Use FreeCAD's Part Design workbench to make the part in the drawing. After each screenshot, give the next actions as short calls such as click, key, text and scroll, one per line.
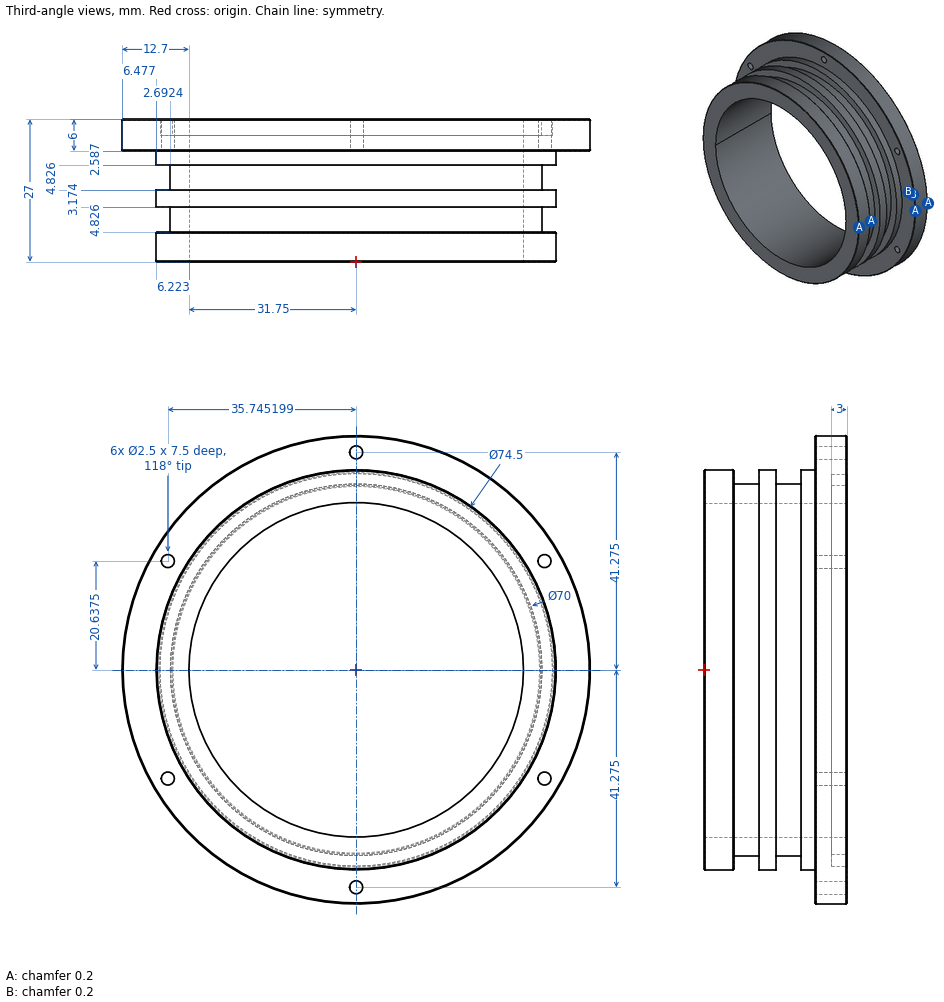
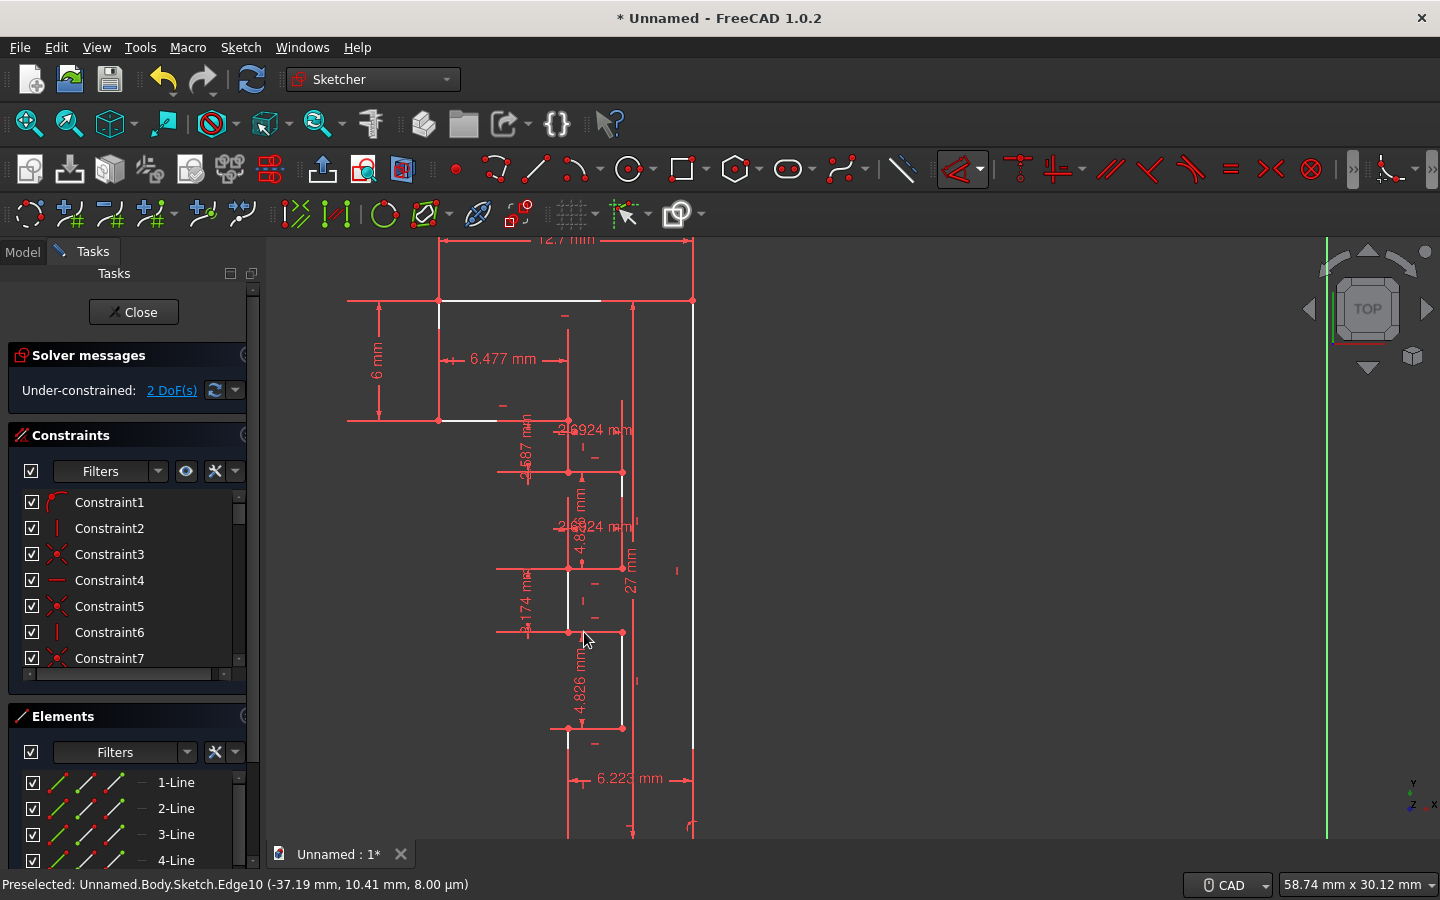
key(l)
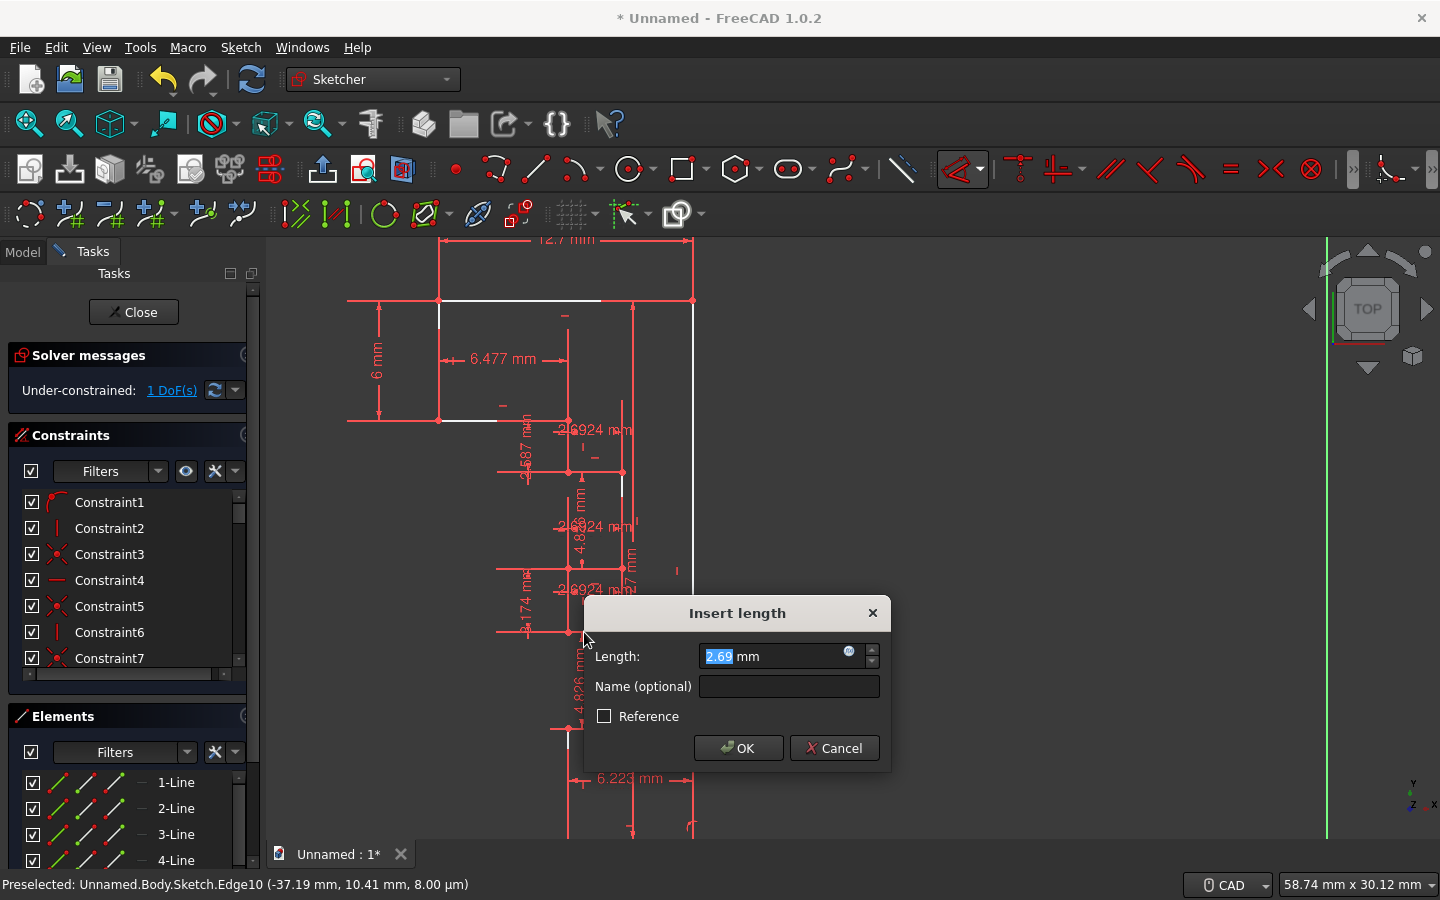
text(2.6924)
key(Return)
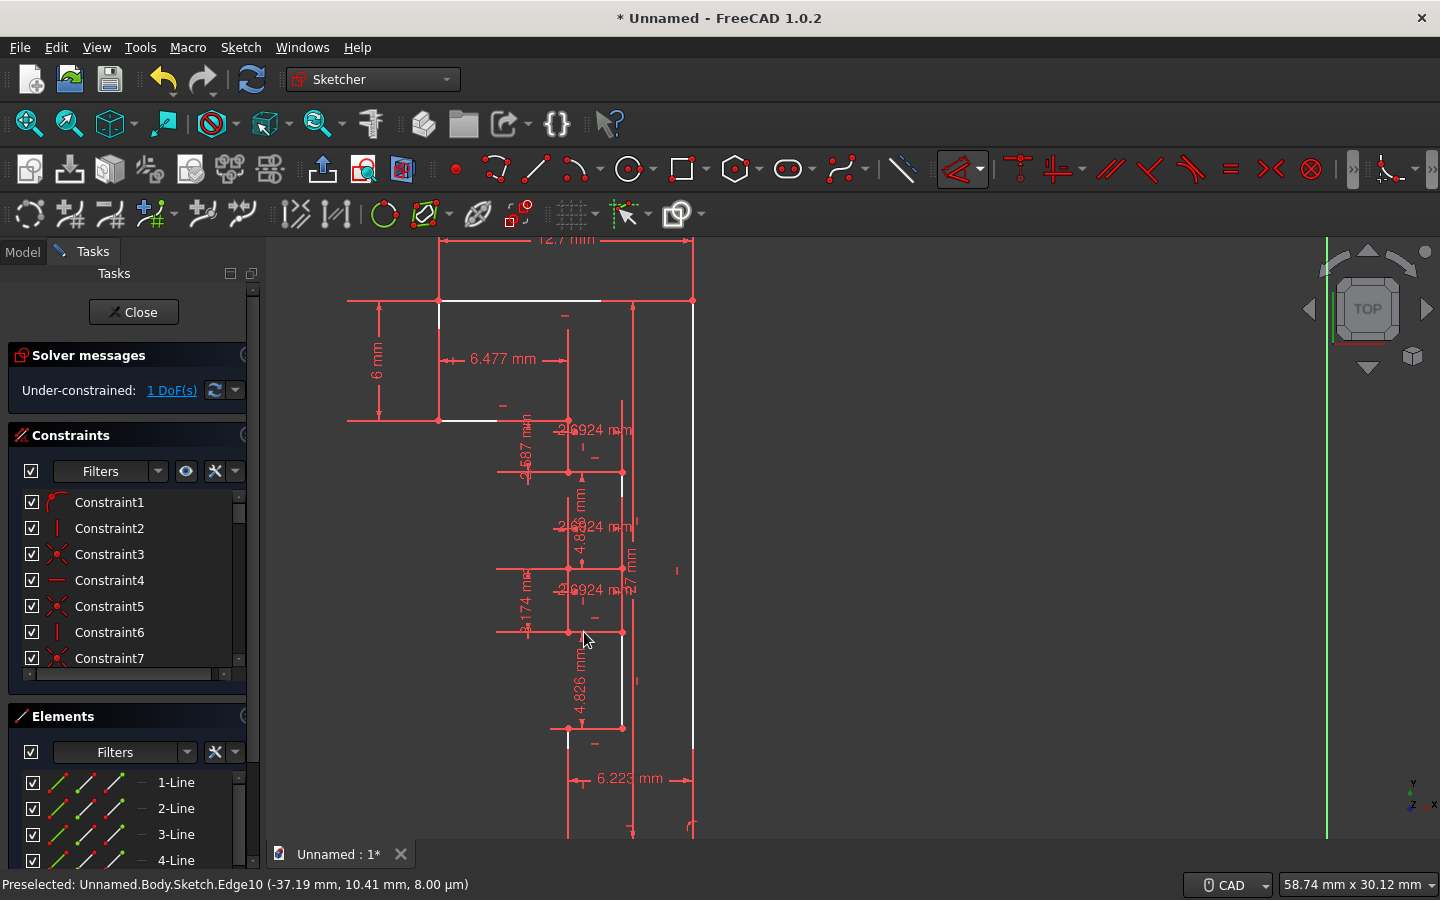
scroll(584, 472, down, 2)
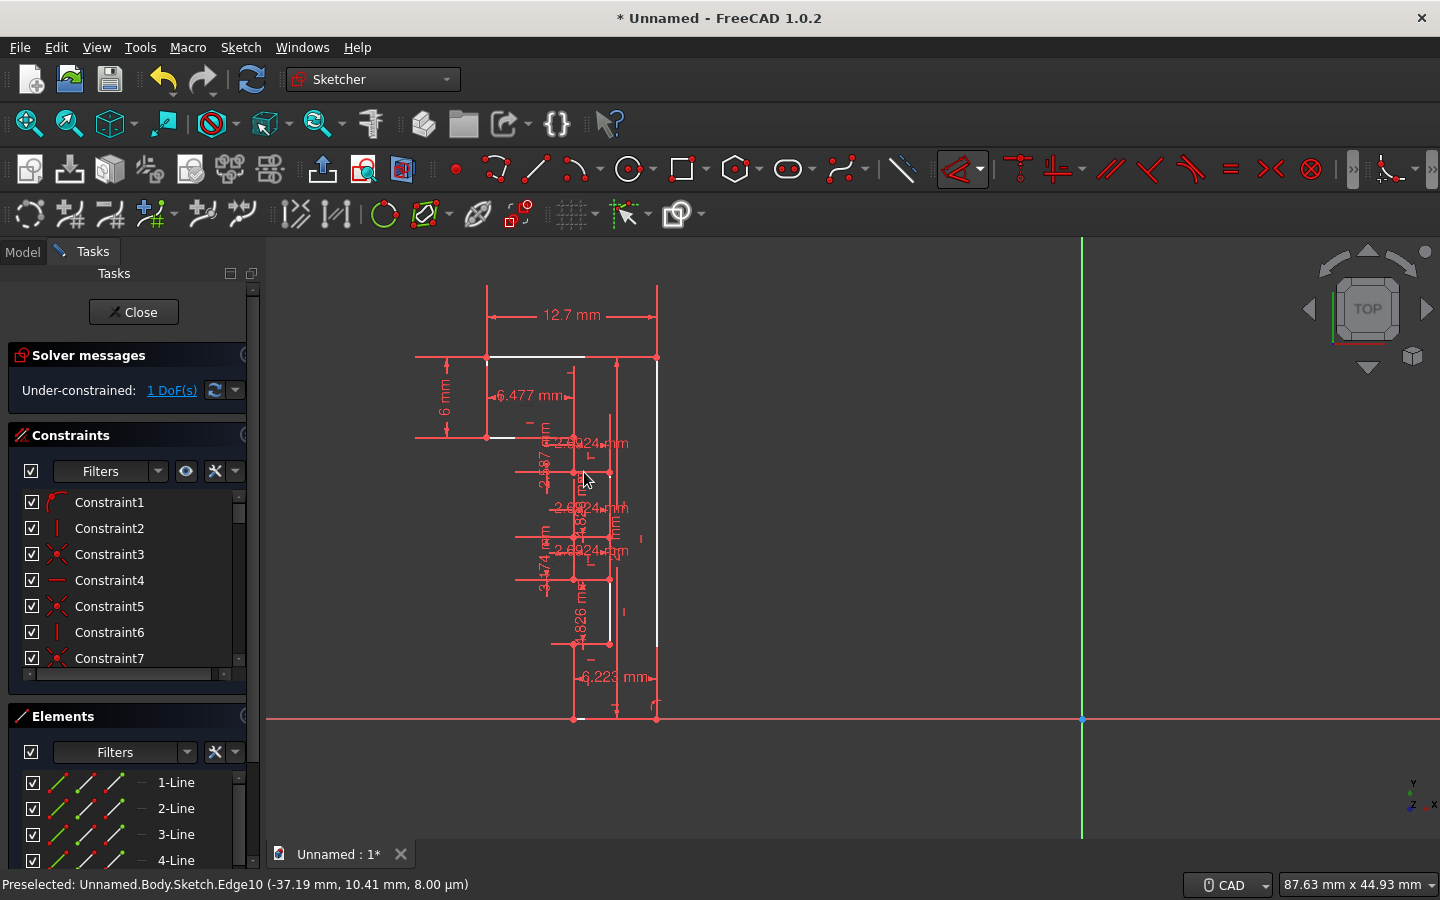
click(657, 719)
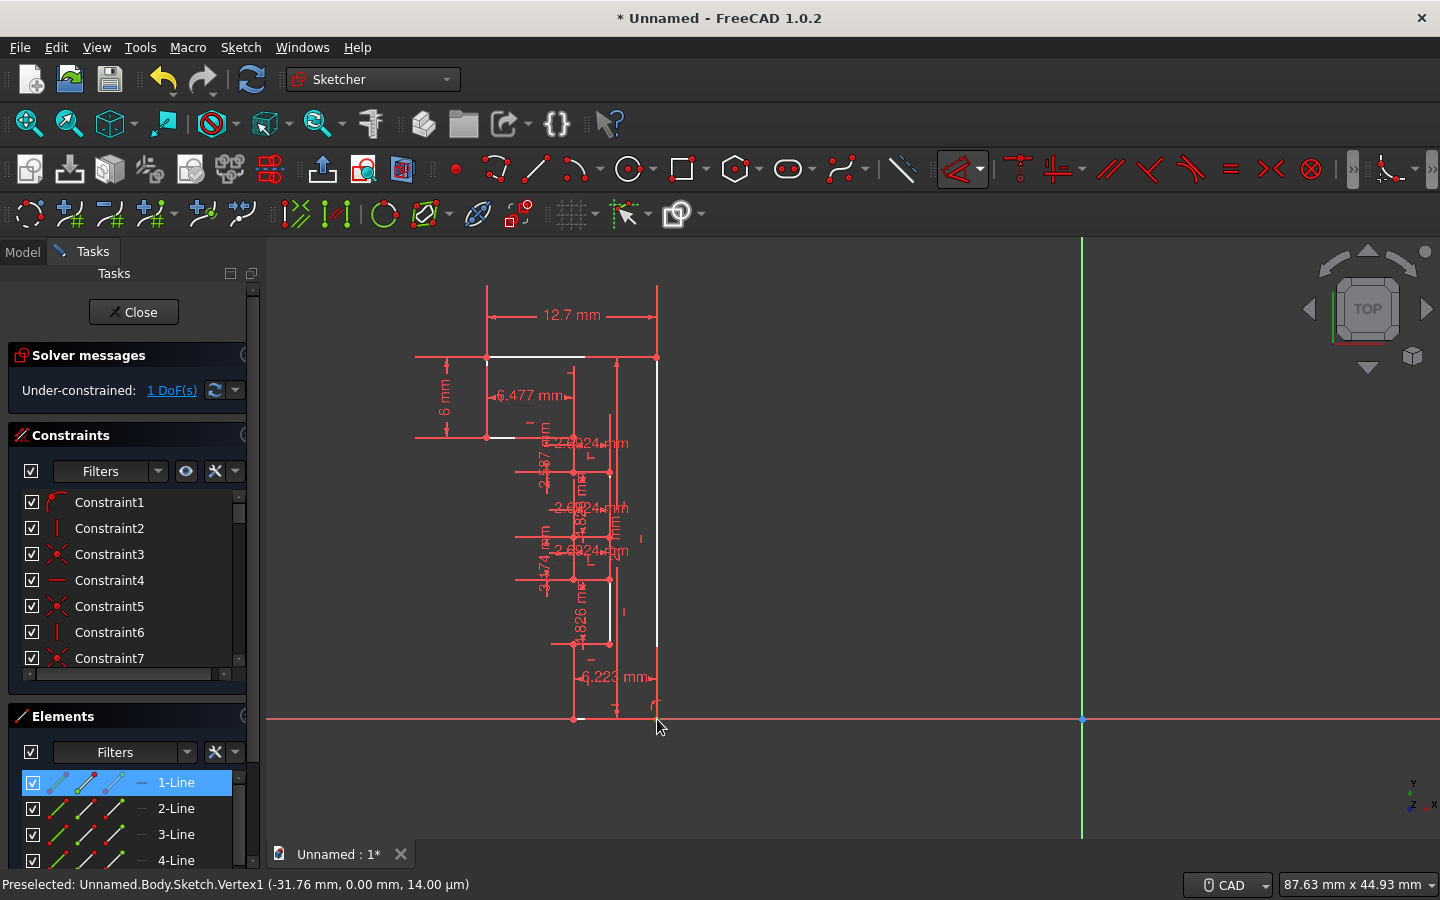
key(l)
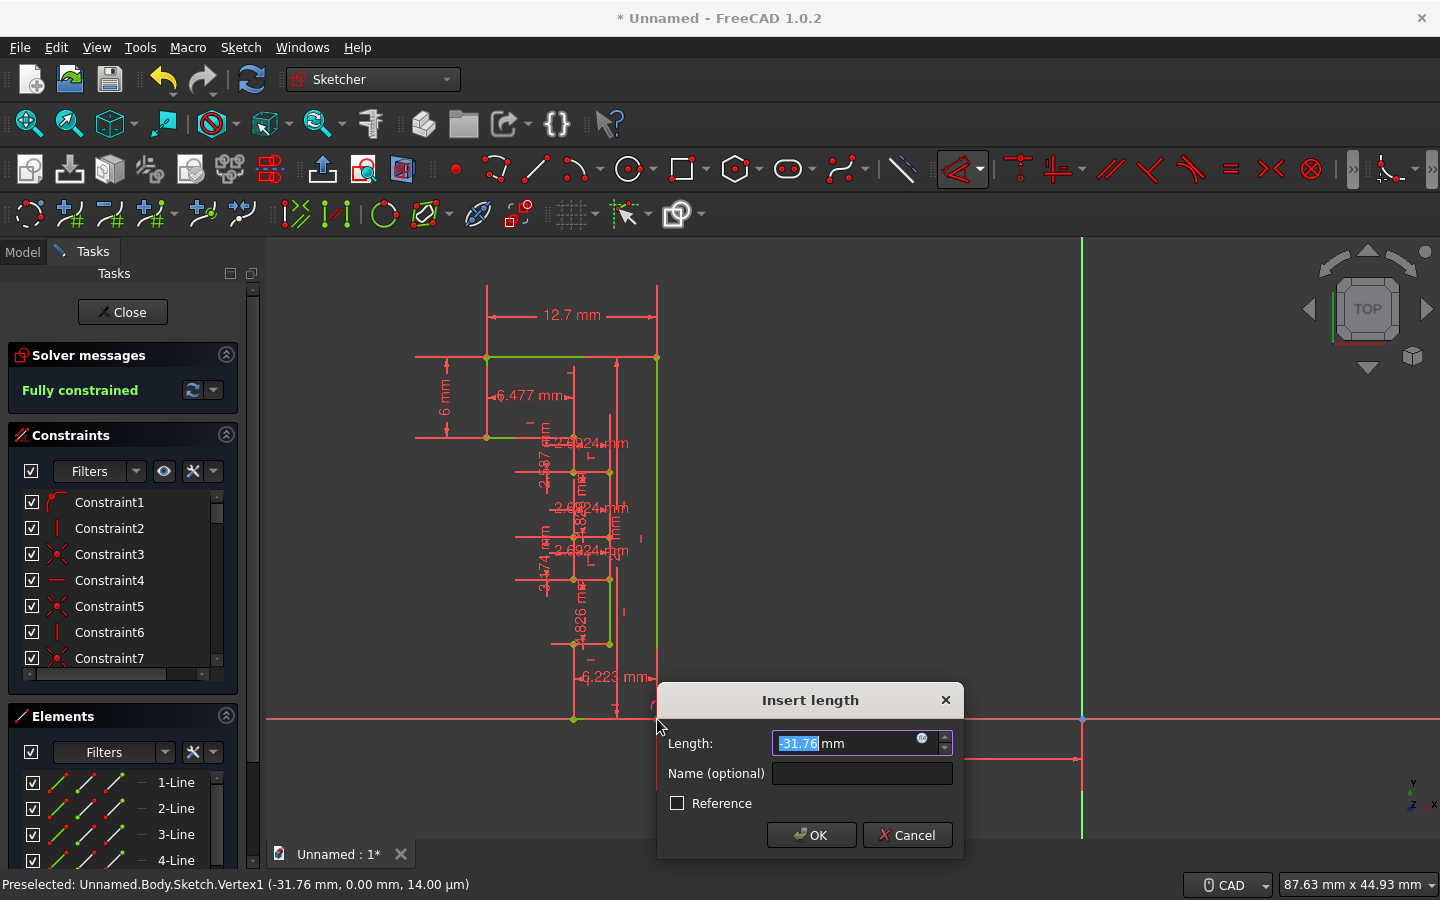
text(-31.75)
key(Return)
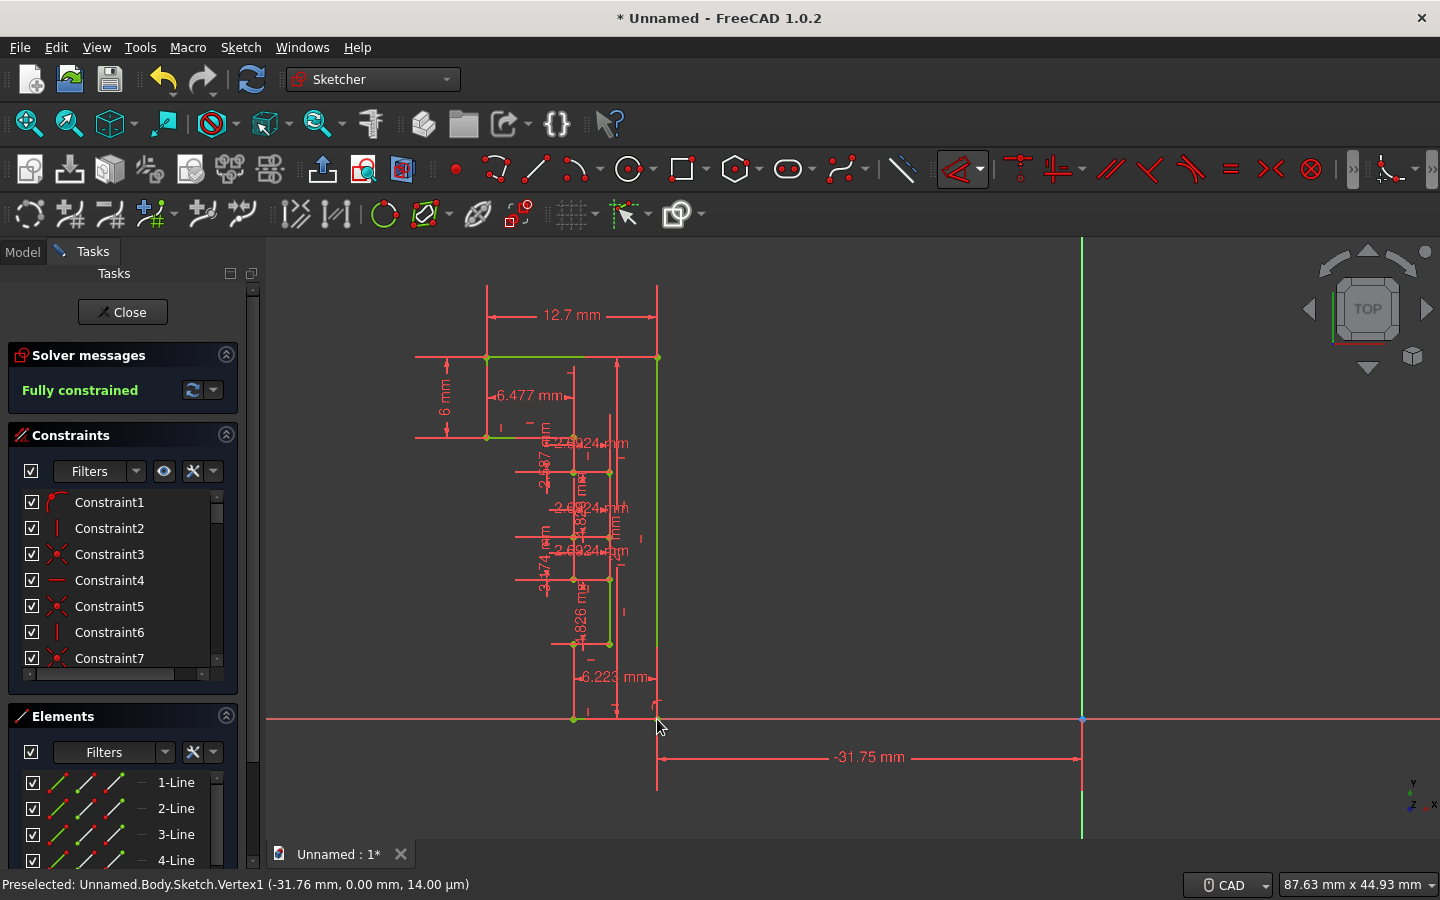
click(123, 312)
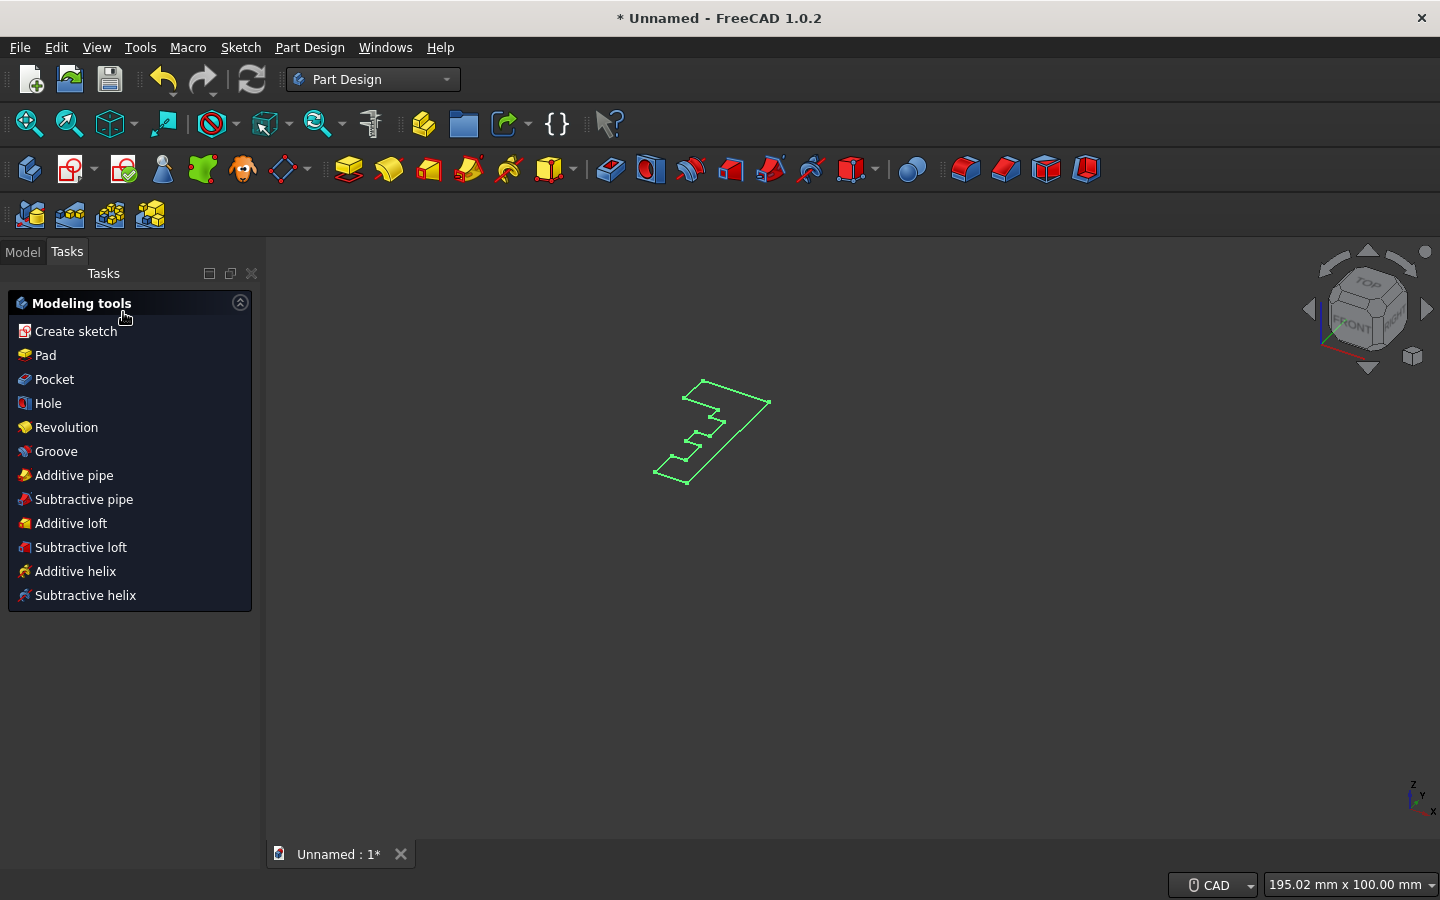
click(390, 170)